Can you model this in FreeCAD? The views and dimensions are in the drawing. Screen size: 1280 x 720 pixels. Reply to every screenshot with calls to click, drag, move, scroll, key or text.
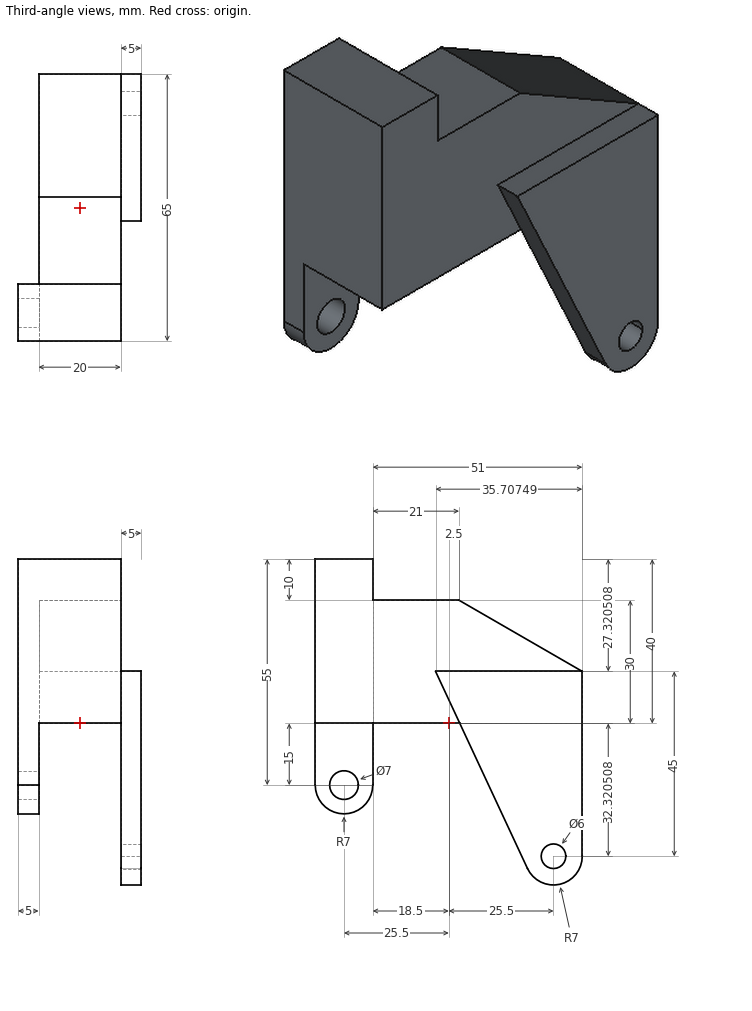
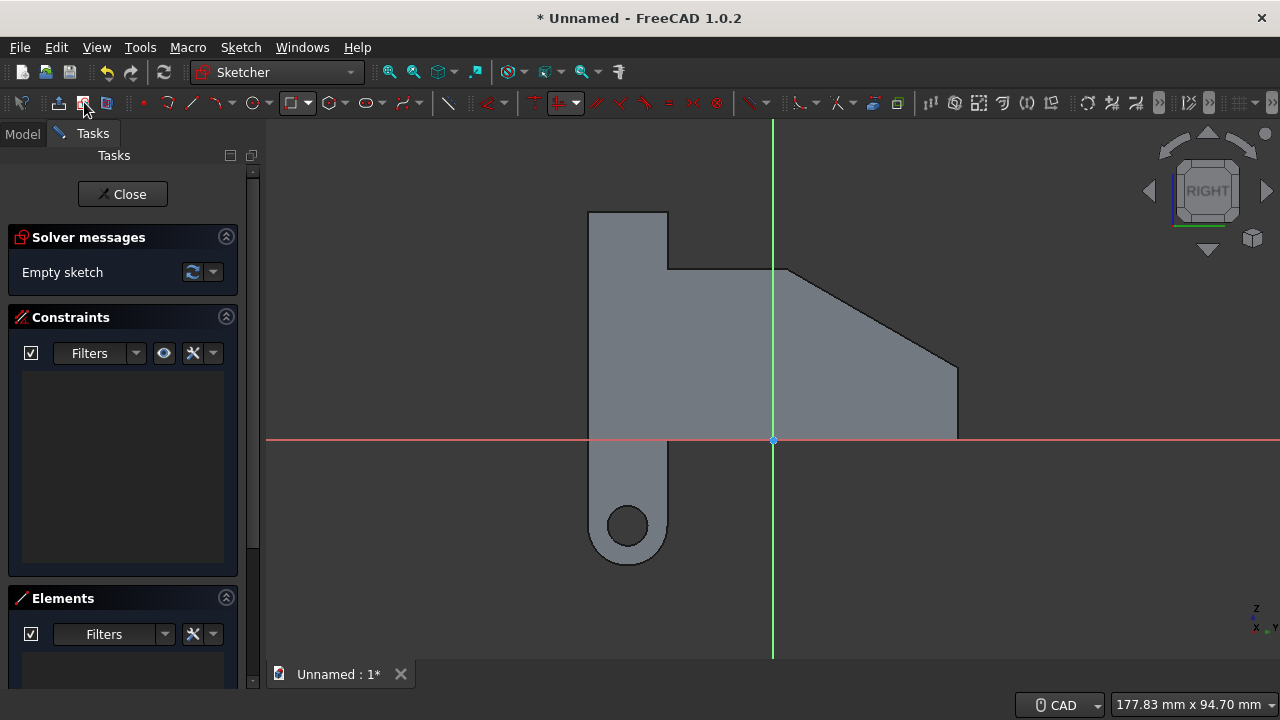
scroll(294, 147, down, 1)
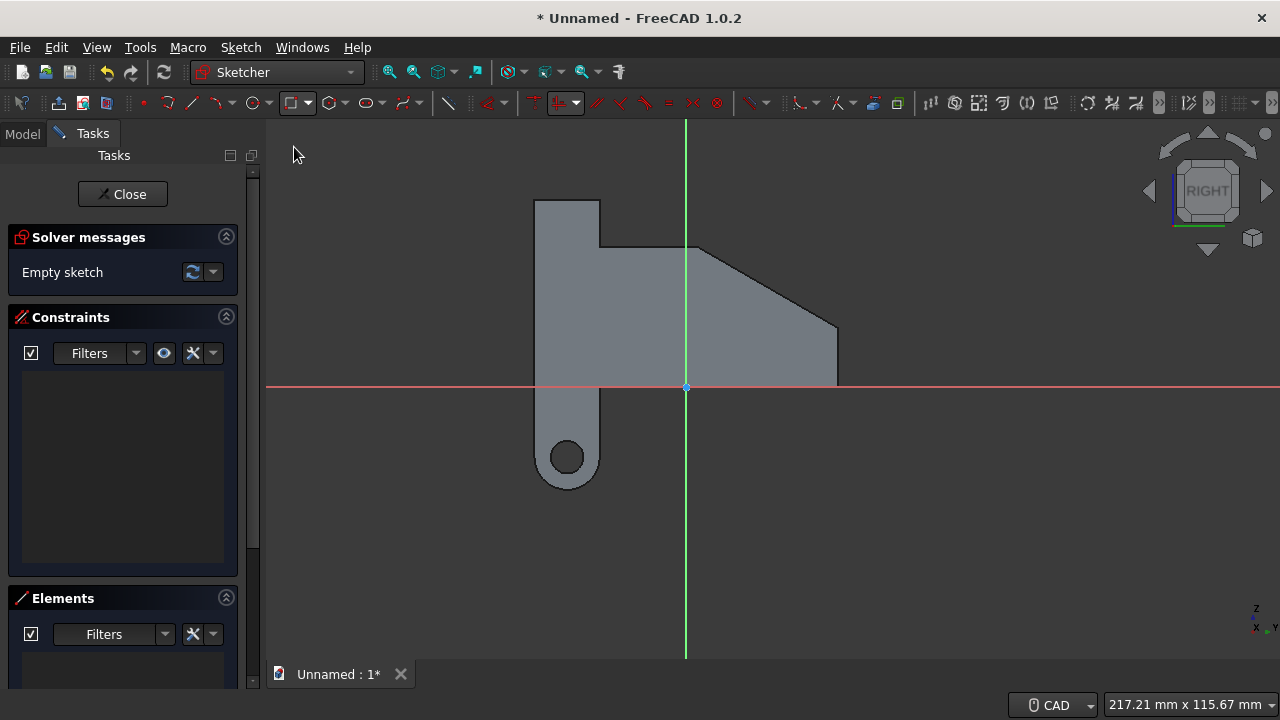
scroll(856, 571, up, 2)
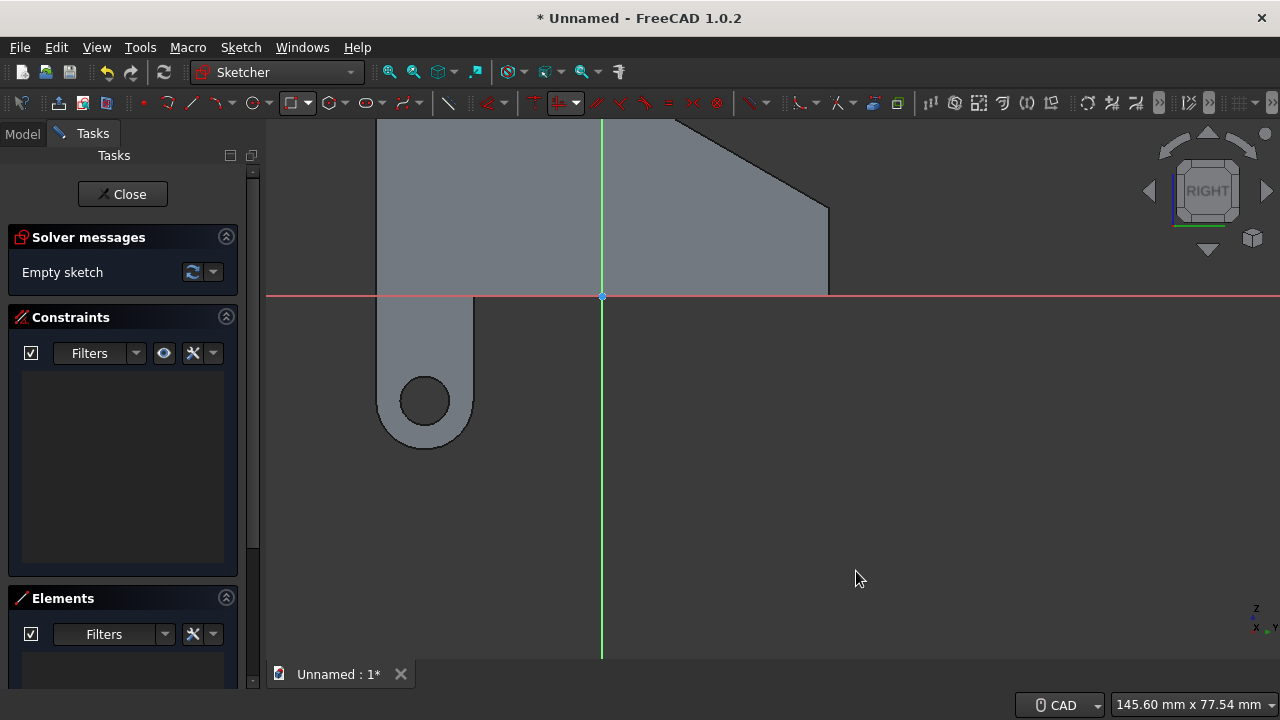
click(168, 104)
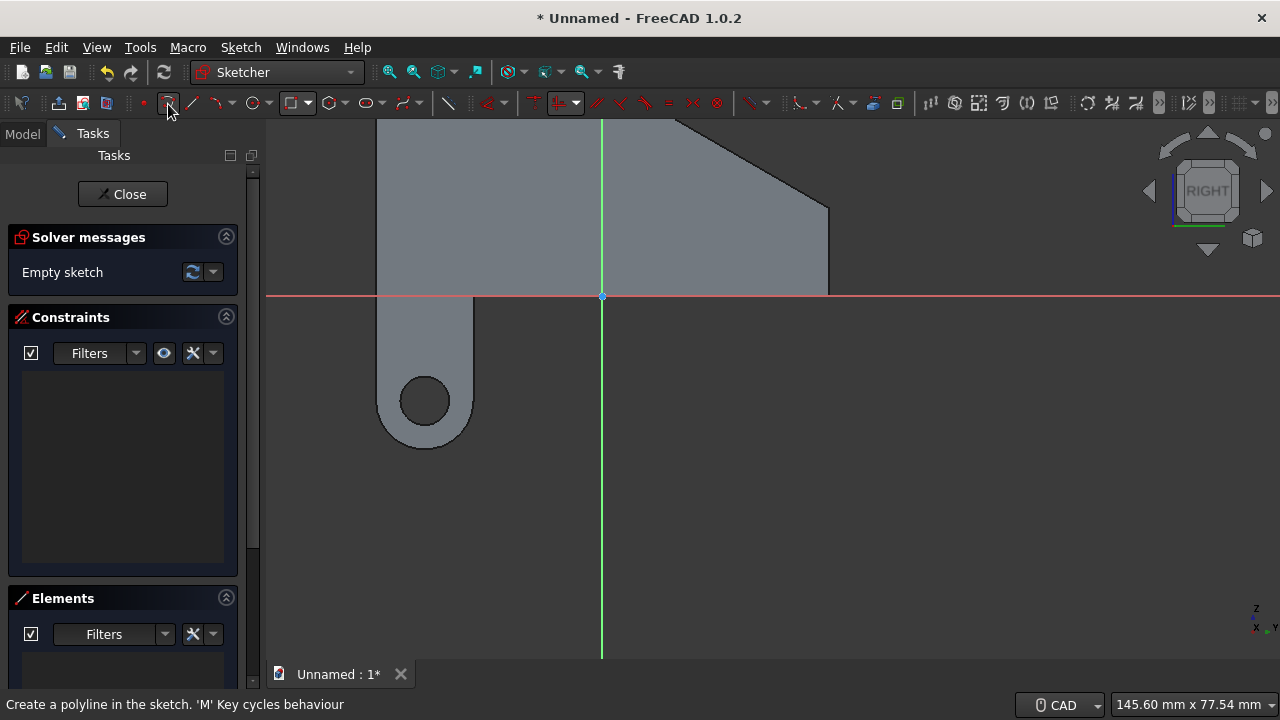
click(829, 521)
click(829, 208)
click(580, 208)
click(736, 542)
right_click(736, 542)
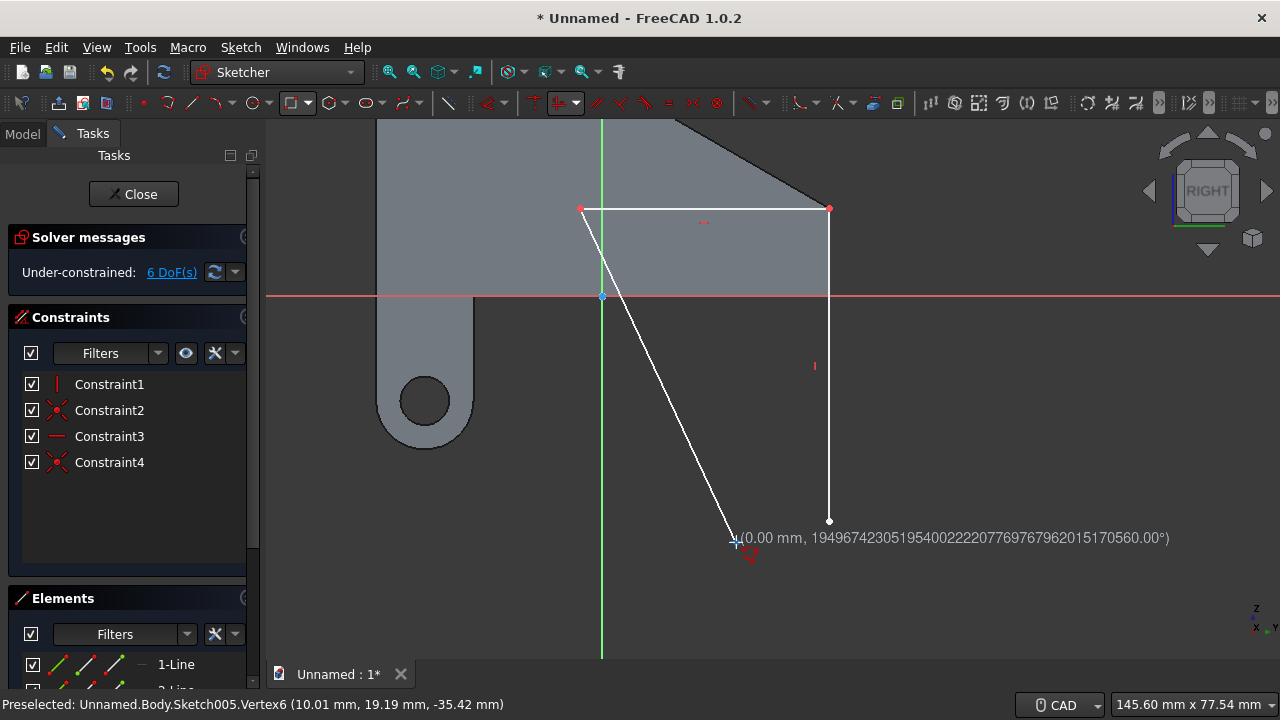
key(g)
key(3)
key(a)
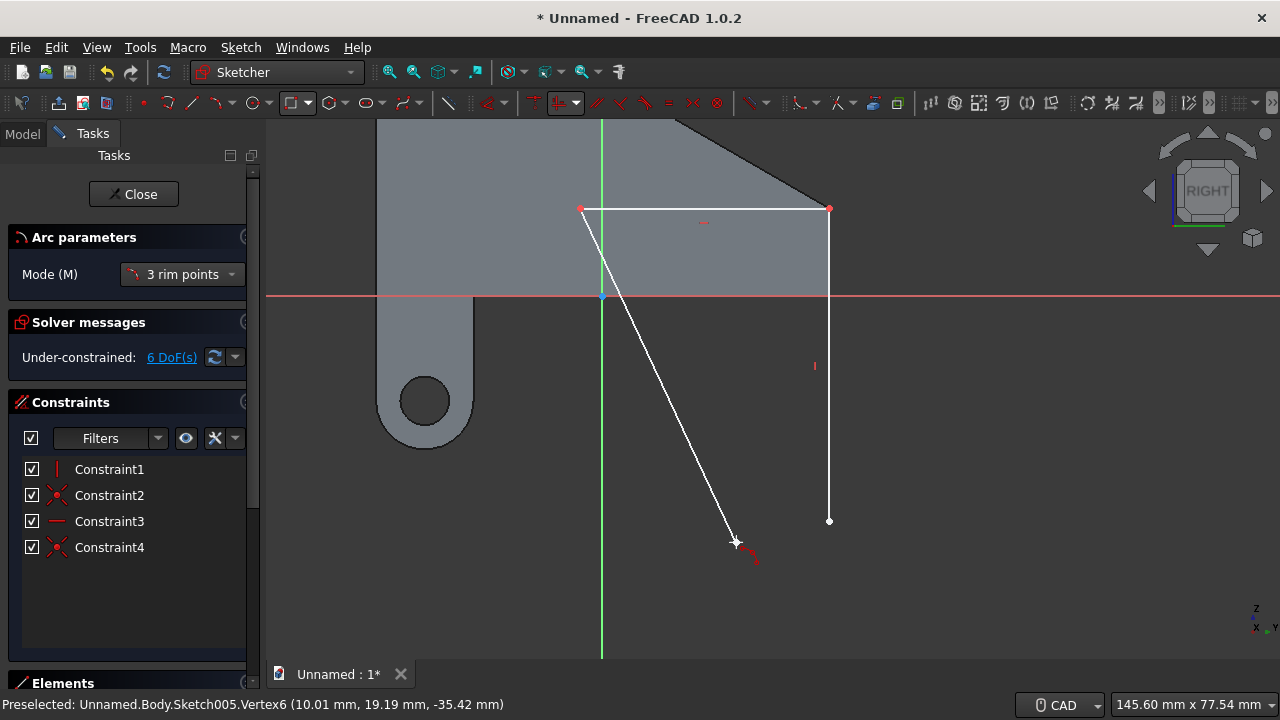
click(736, 543)
click(829, 522)
click(791, 569)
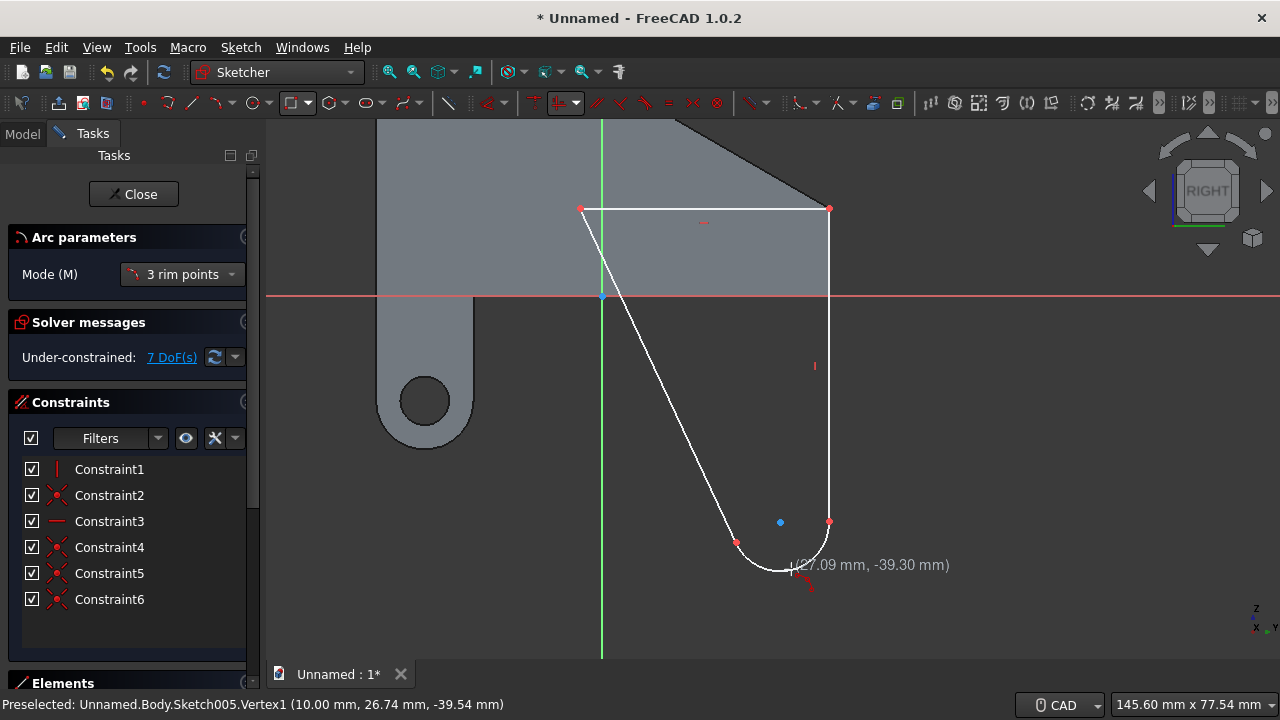
key(g)
key(c)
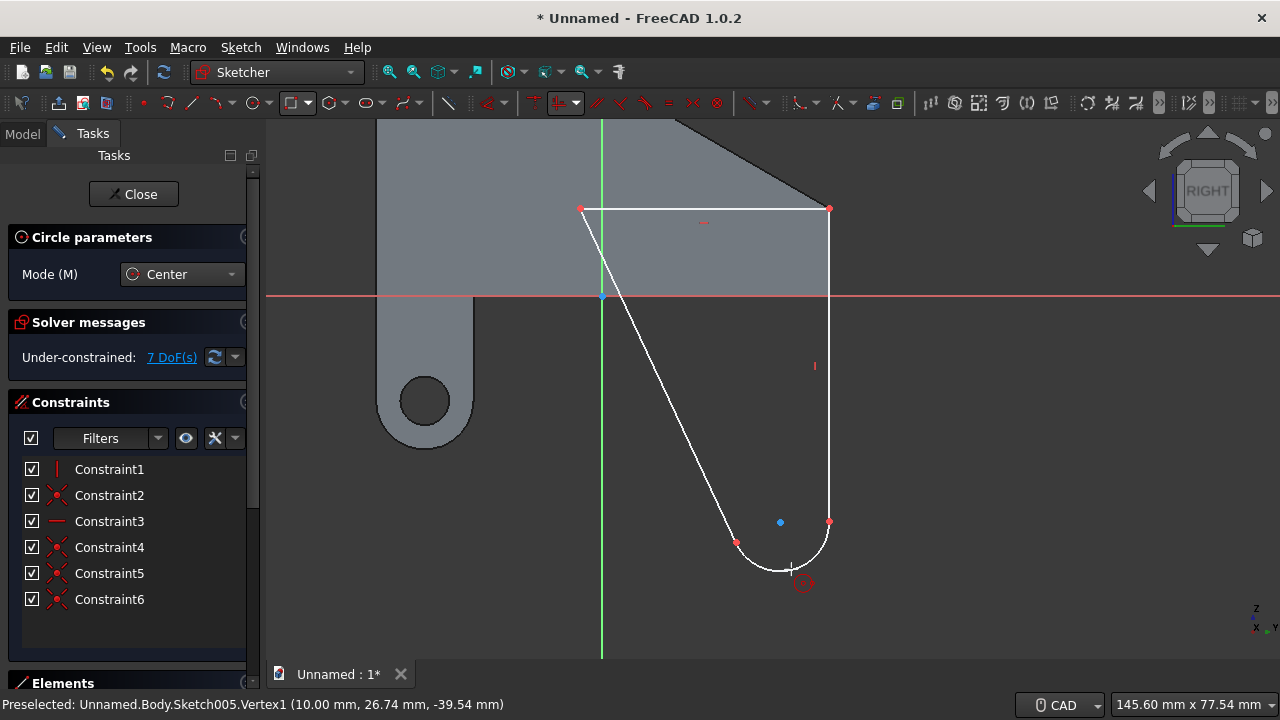
click(780, 521)
move(795, 507)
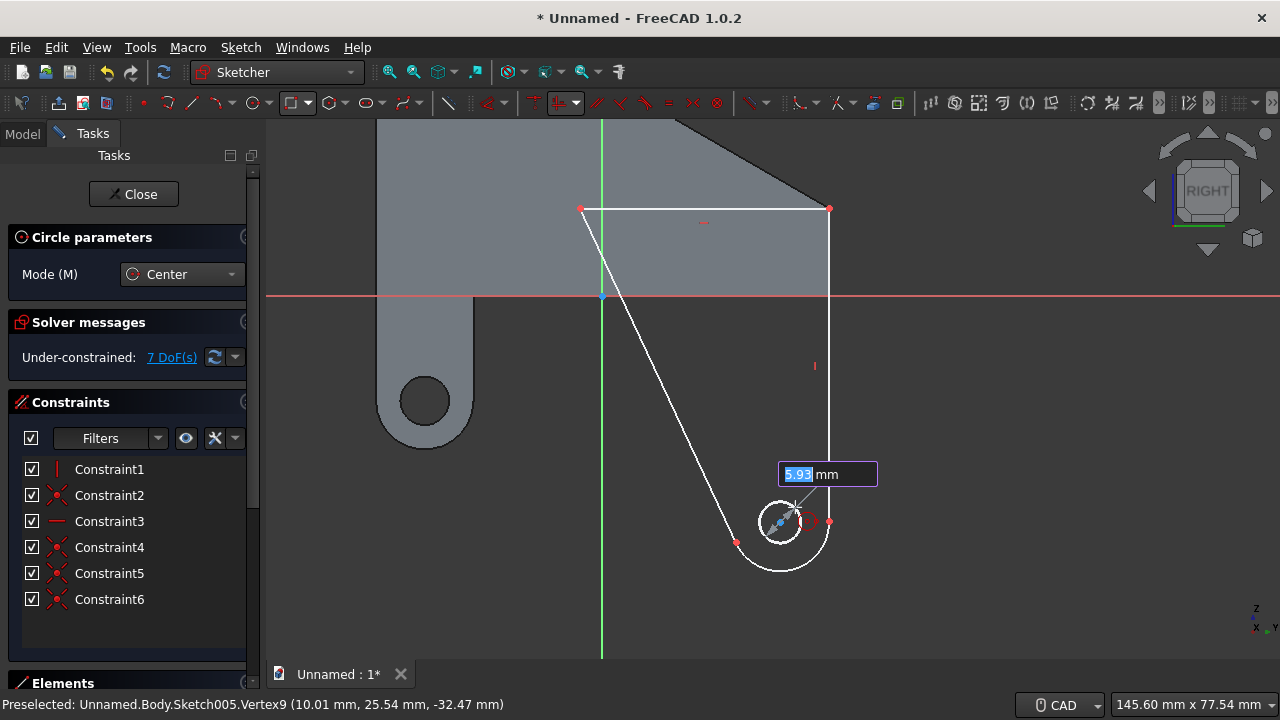
text(6)
key(Return)
key(Escape)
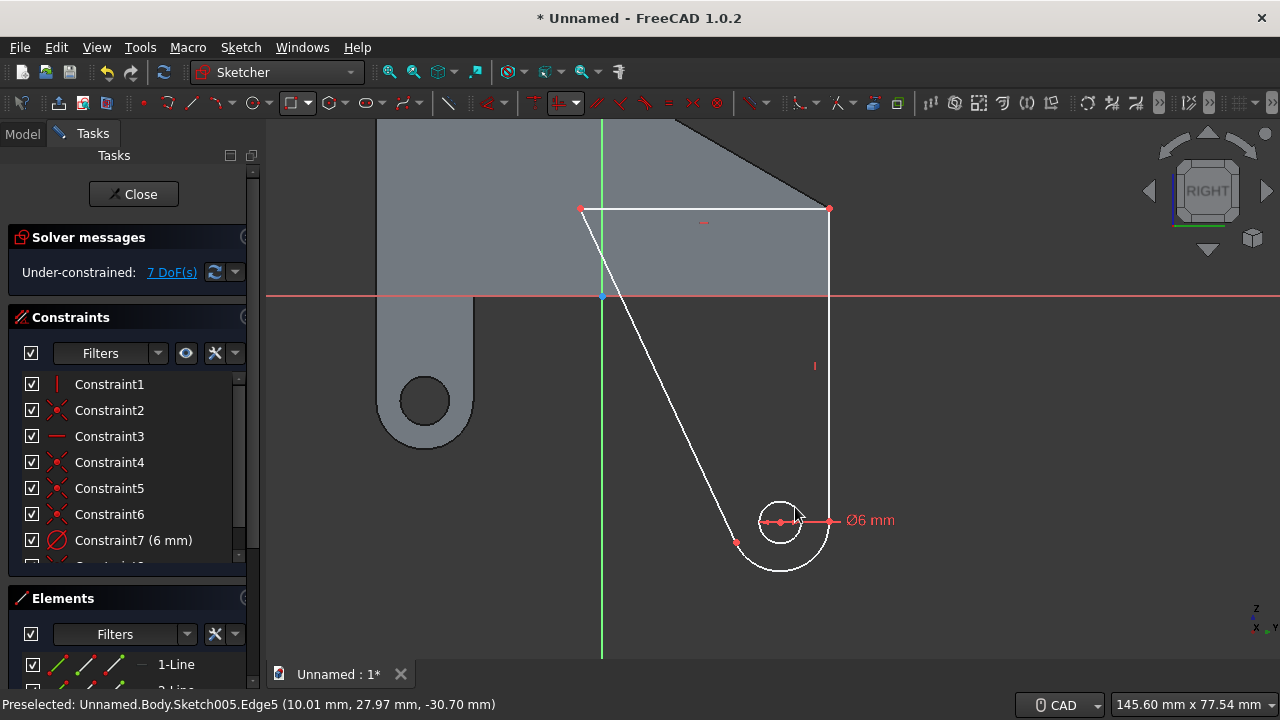
click(829, 428)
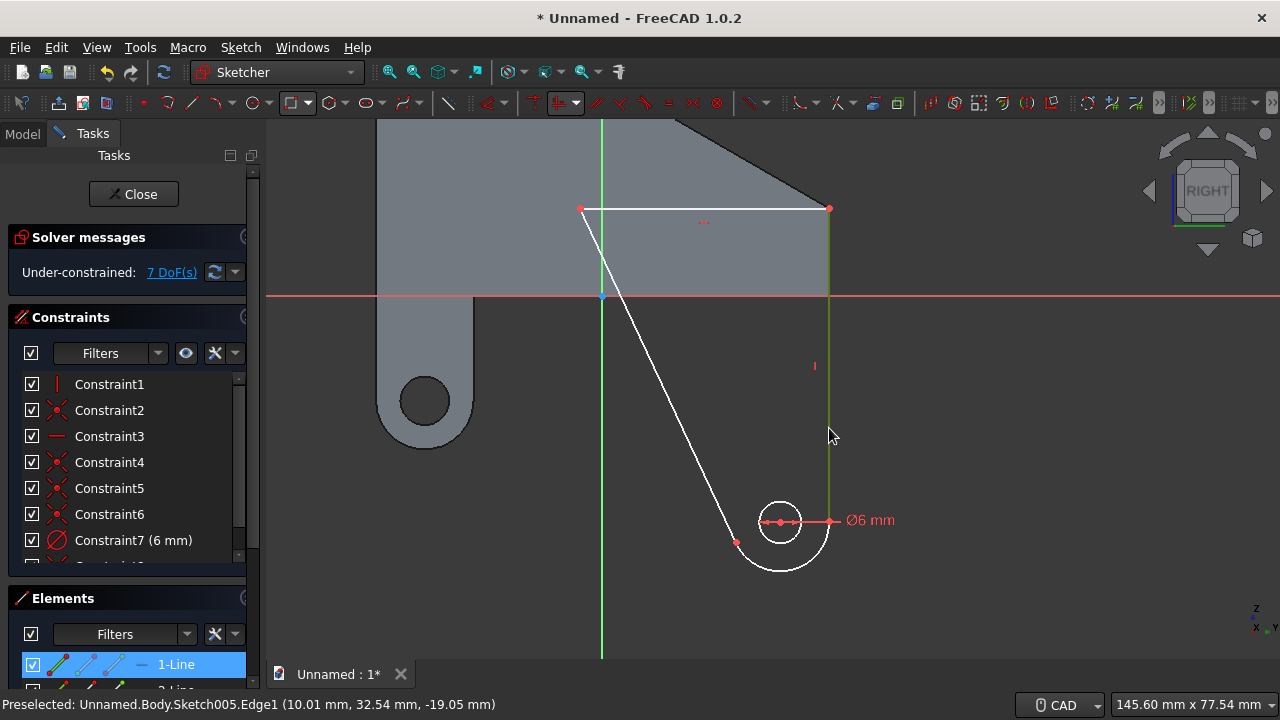
click(765, 569)